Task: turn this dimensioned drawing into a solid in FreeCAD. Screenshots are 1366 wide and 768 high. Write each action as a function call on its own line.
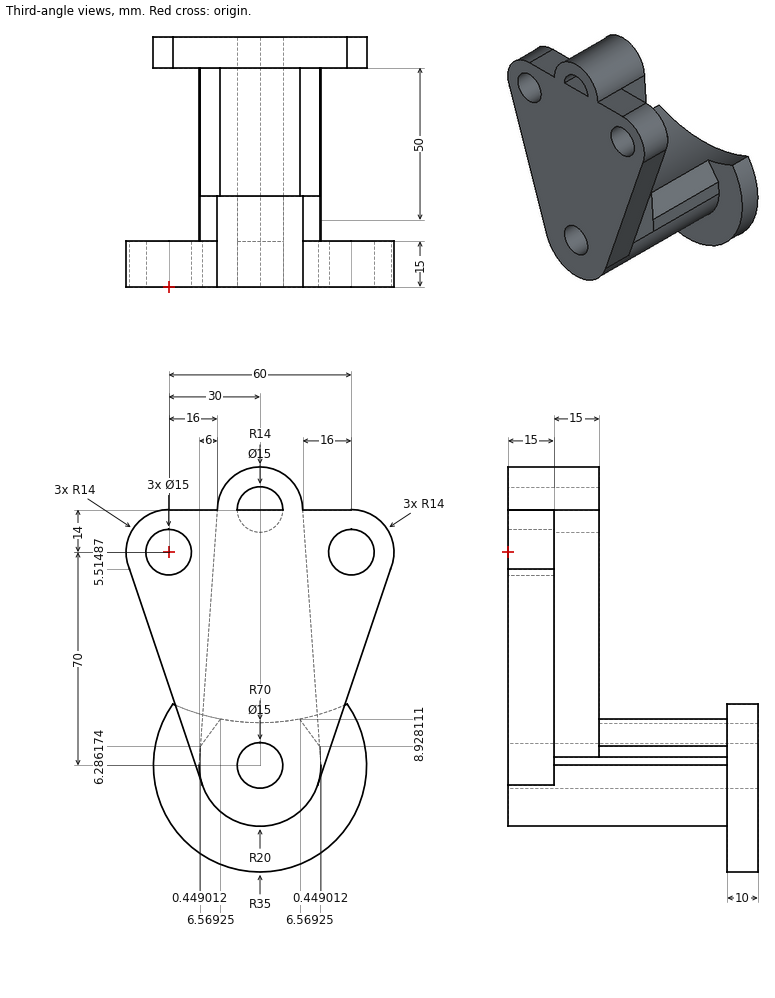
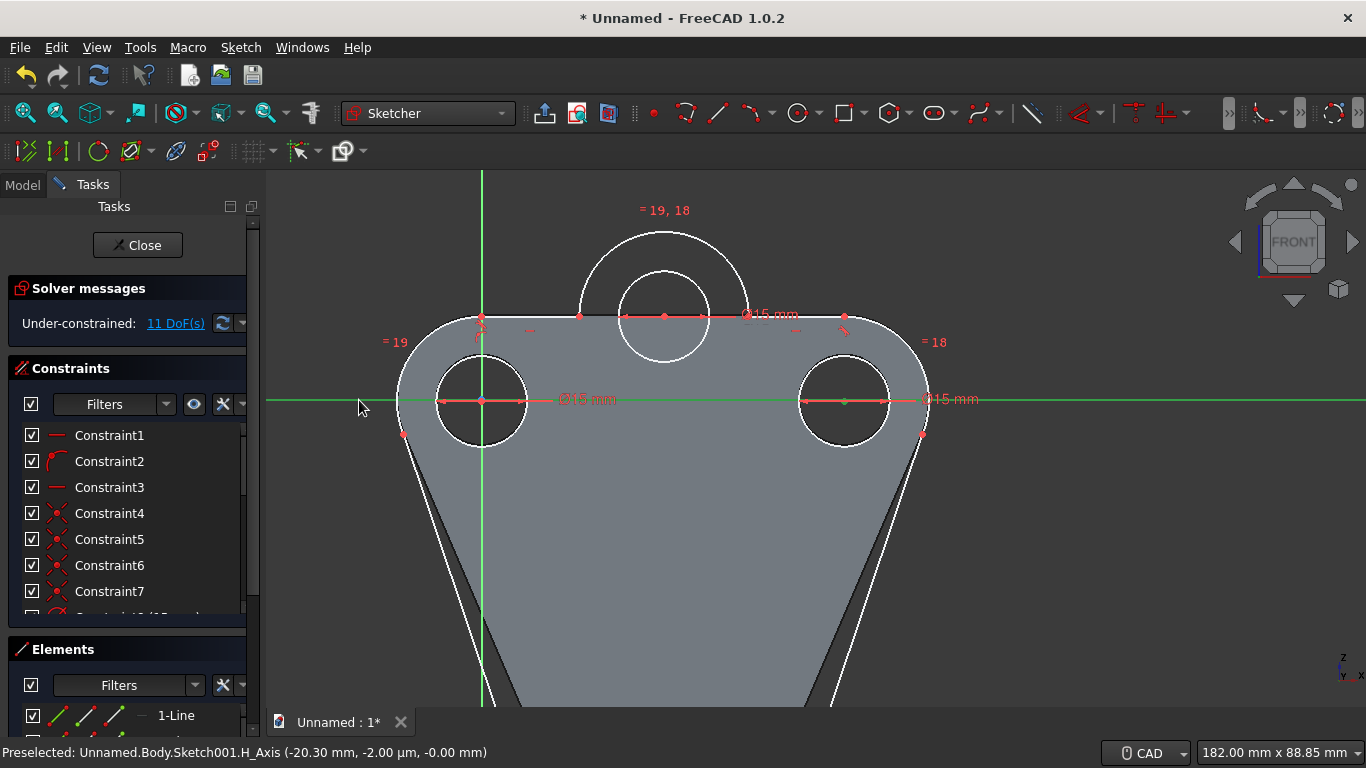
click(1134, 114)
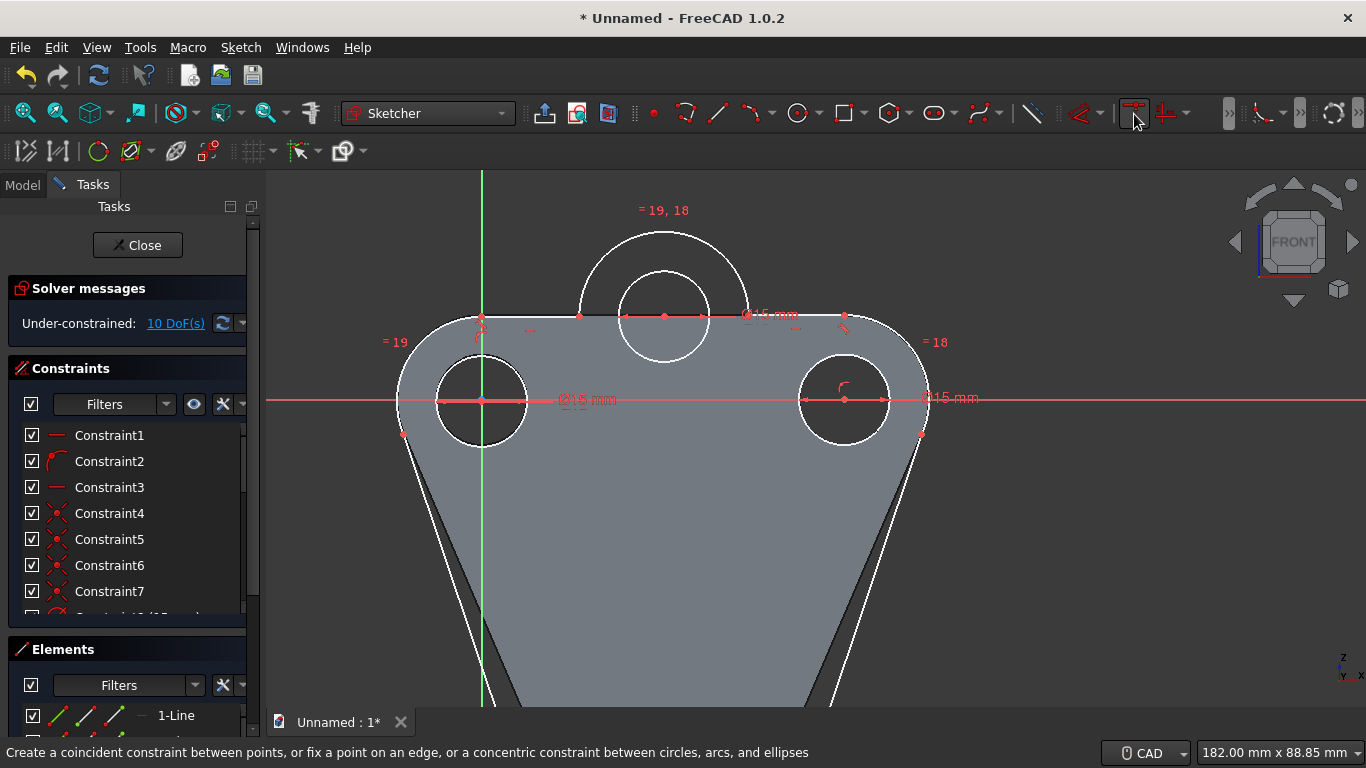
click(482, 402)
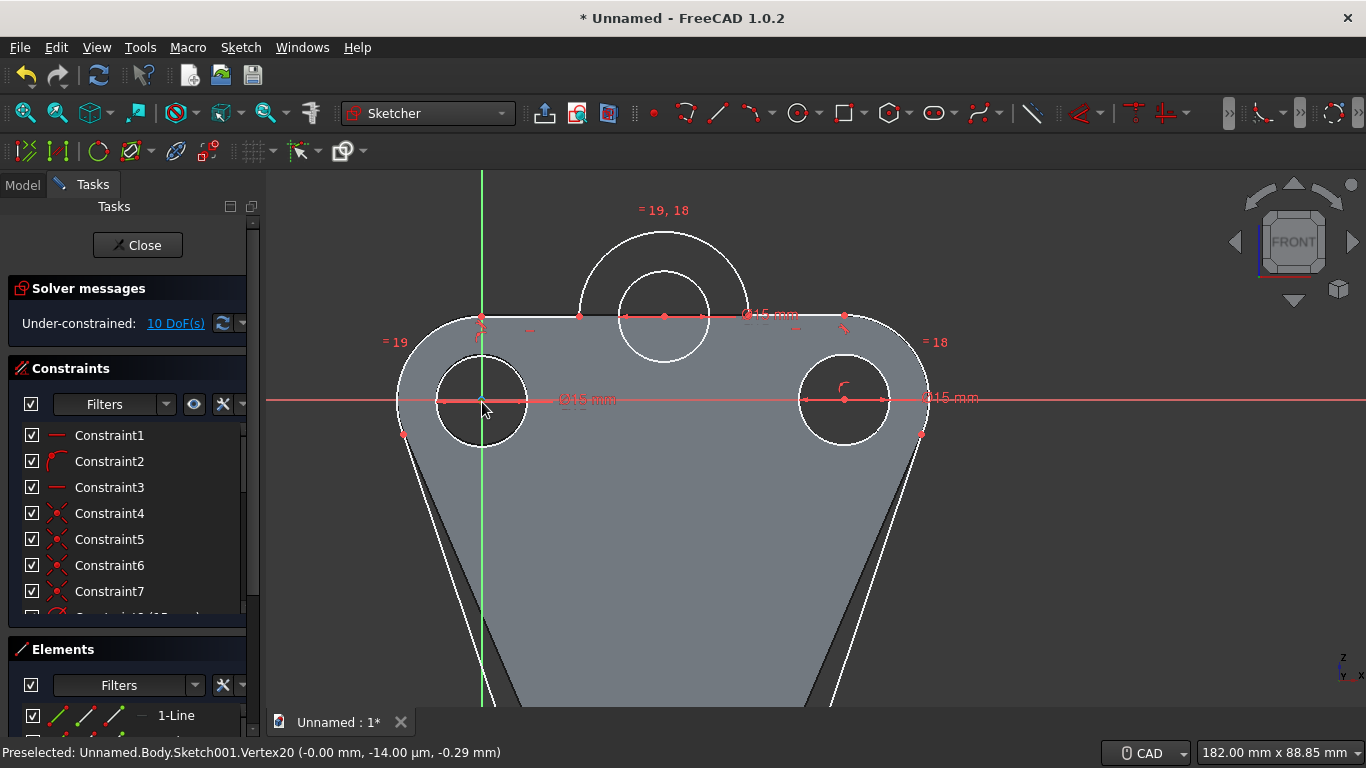
click(359, 400)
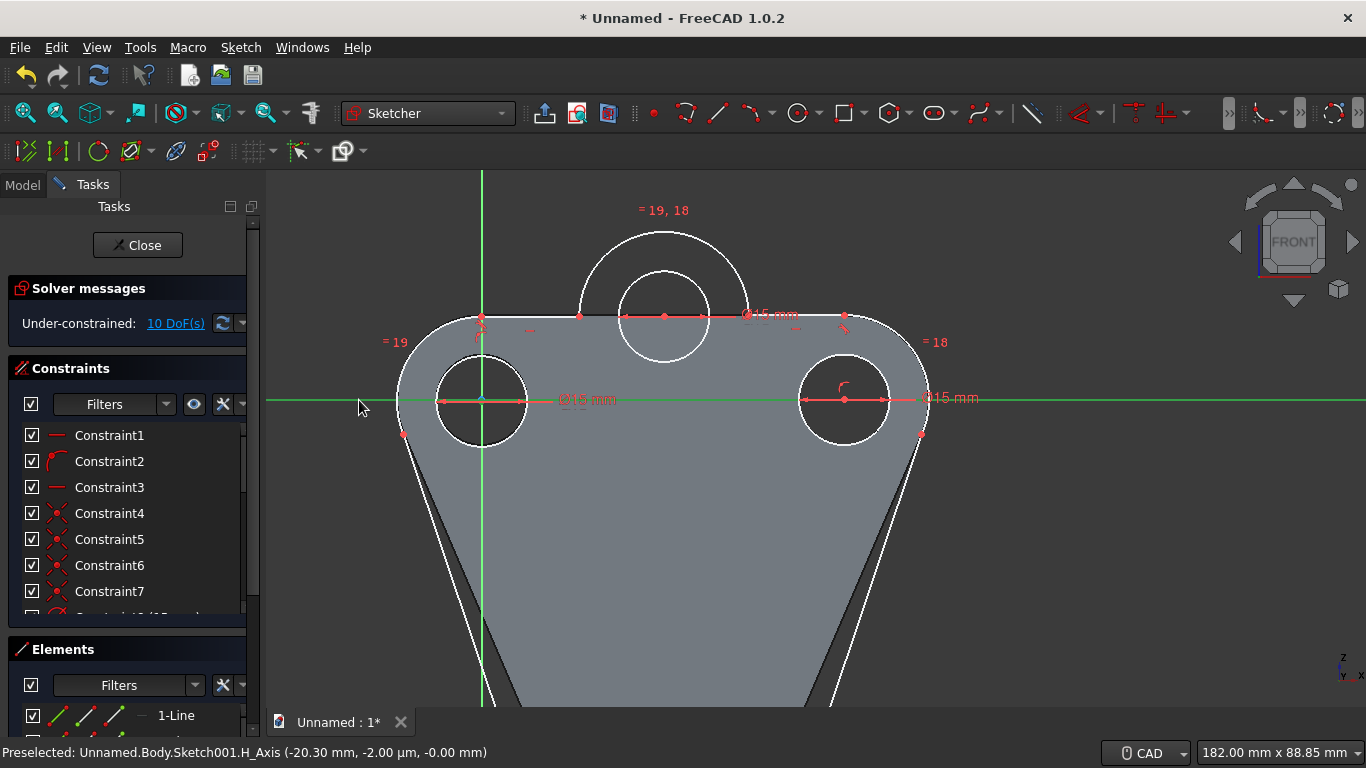
click(1134, 114)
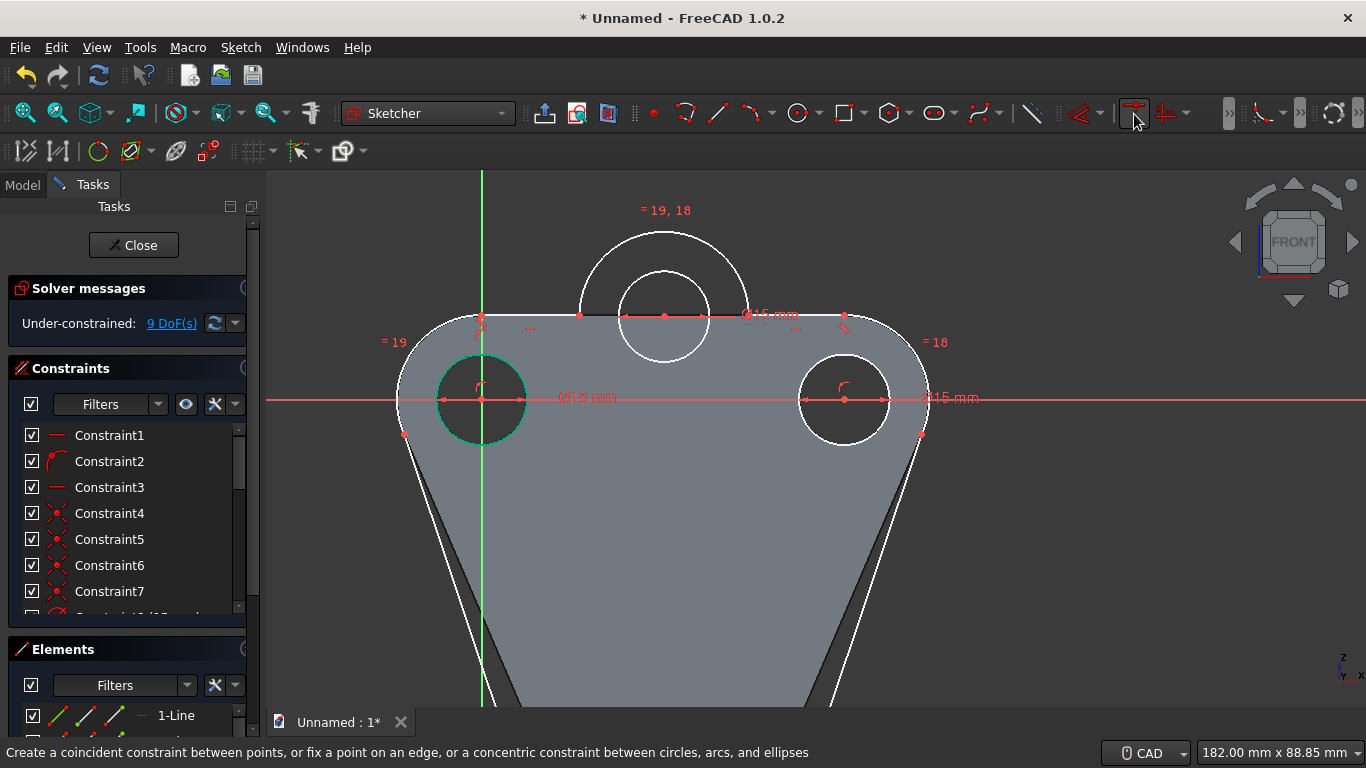
click(1080, 114)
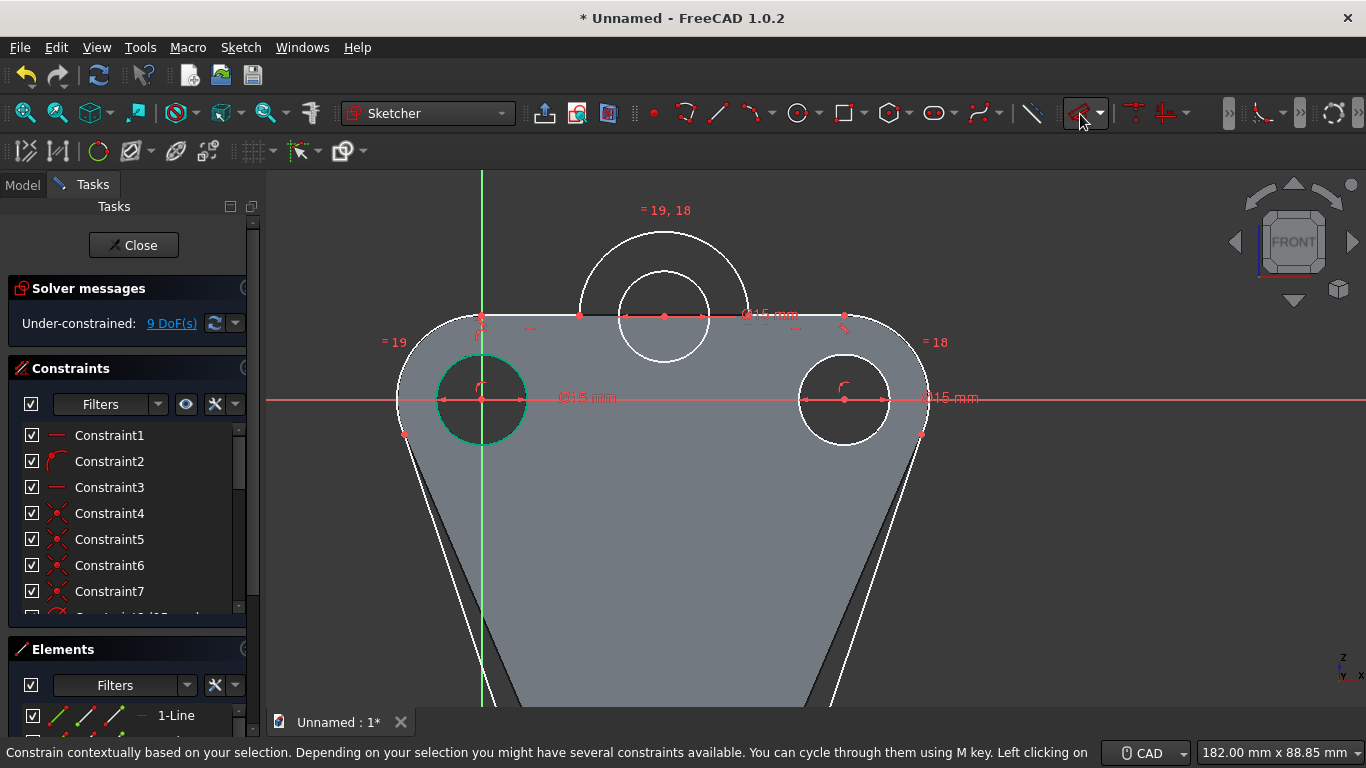
scroll(816, 317, down, 4)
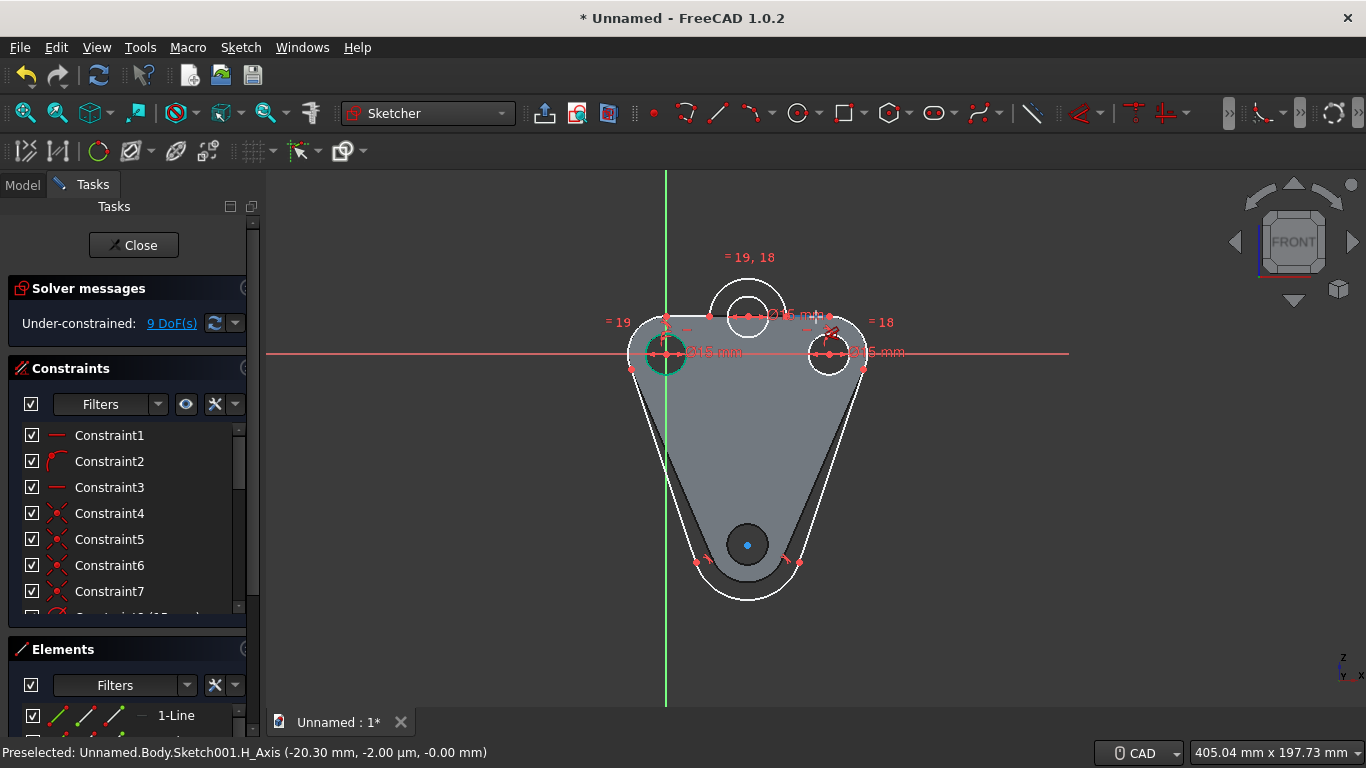
click(722, 593)
click(707, 621)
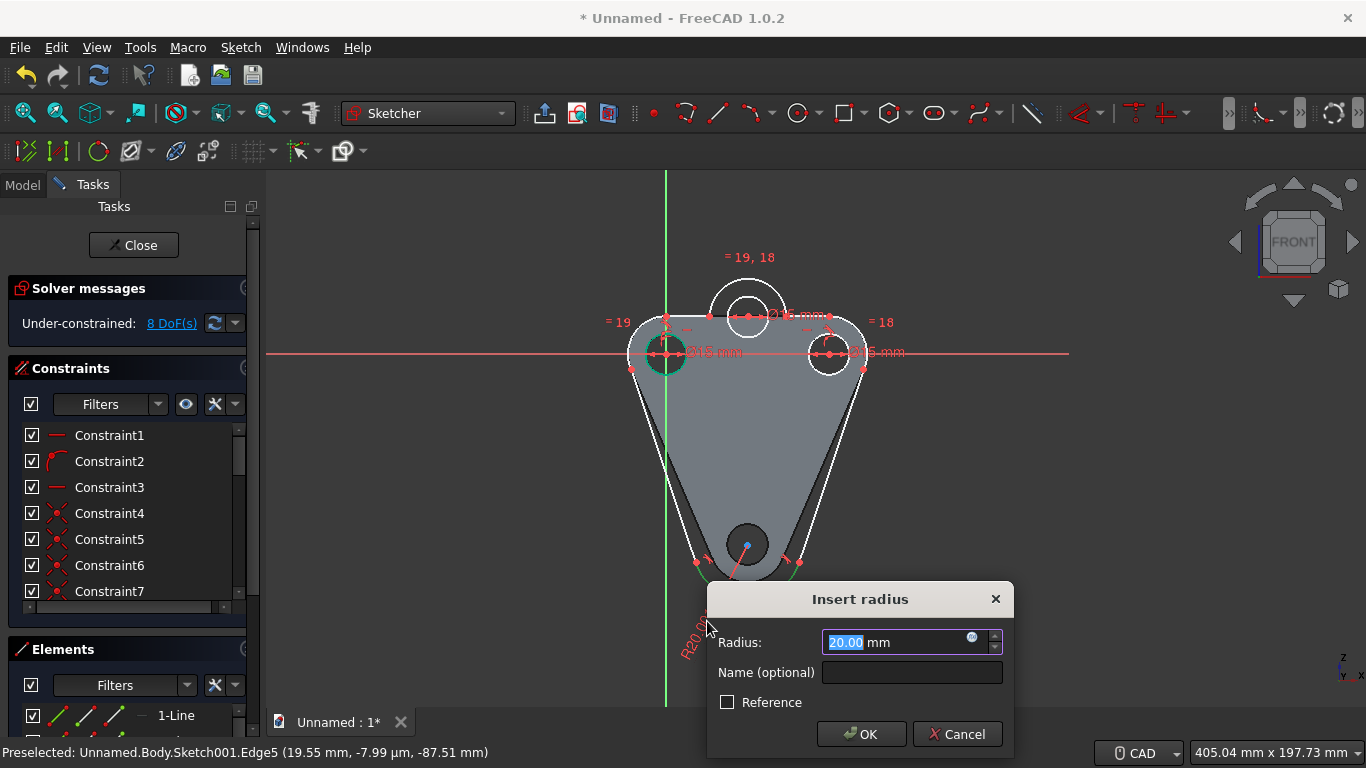
text(20)
key(Return)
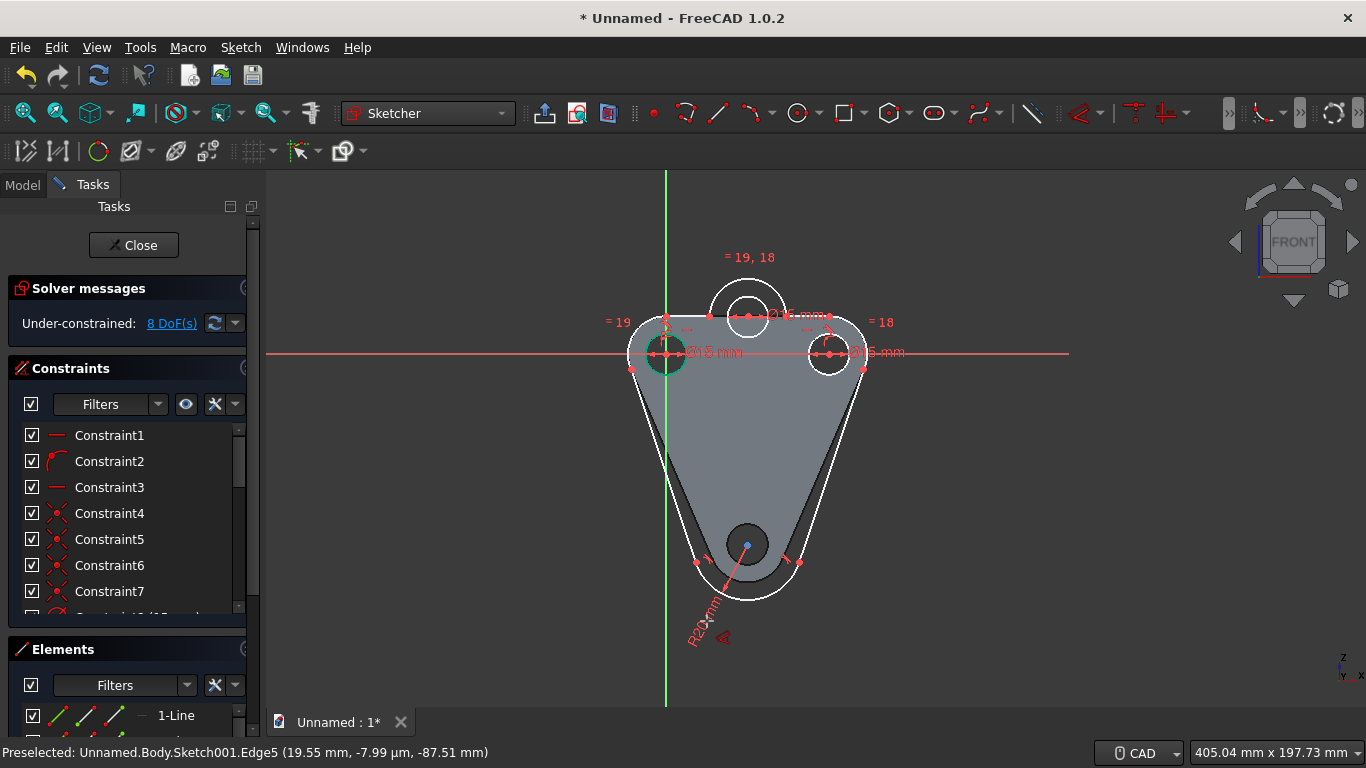
click(850, 323)
click(868, 296)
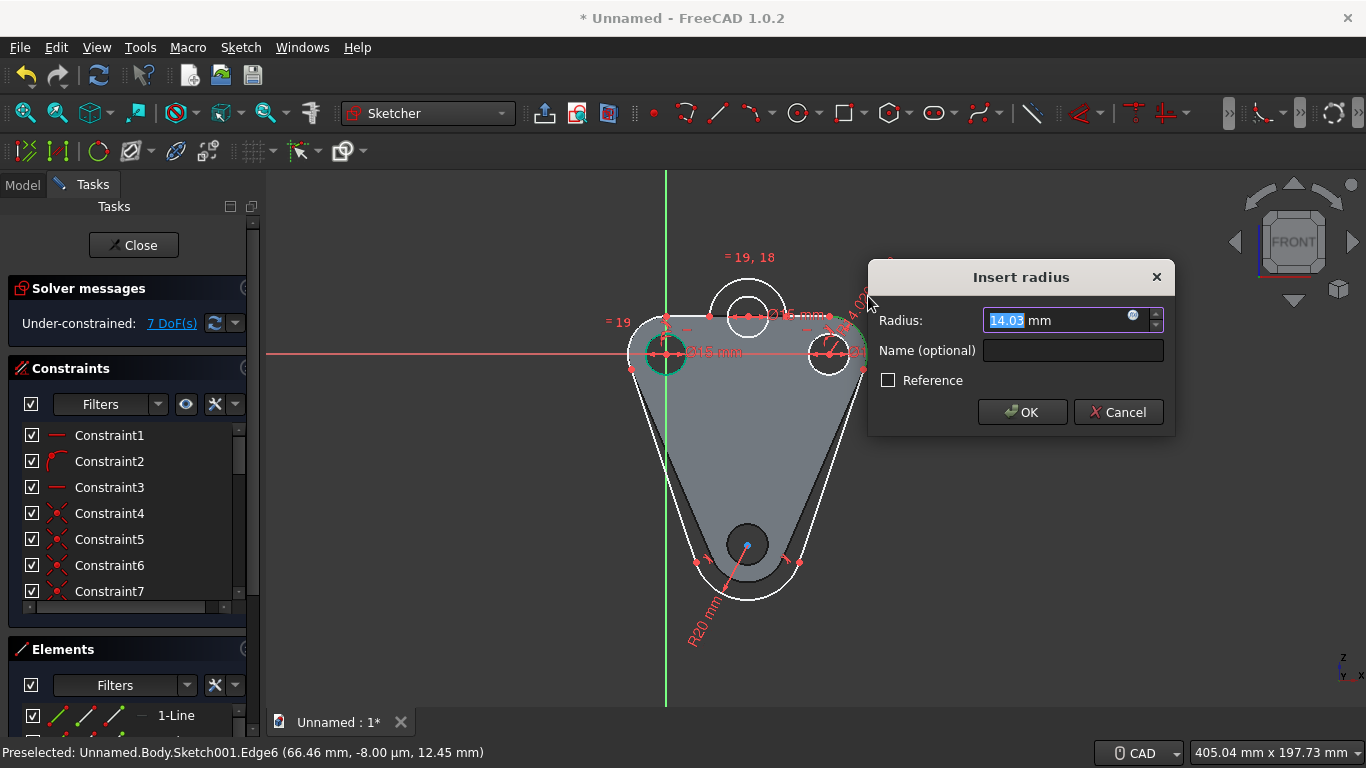
text(14)
key(Return)